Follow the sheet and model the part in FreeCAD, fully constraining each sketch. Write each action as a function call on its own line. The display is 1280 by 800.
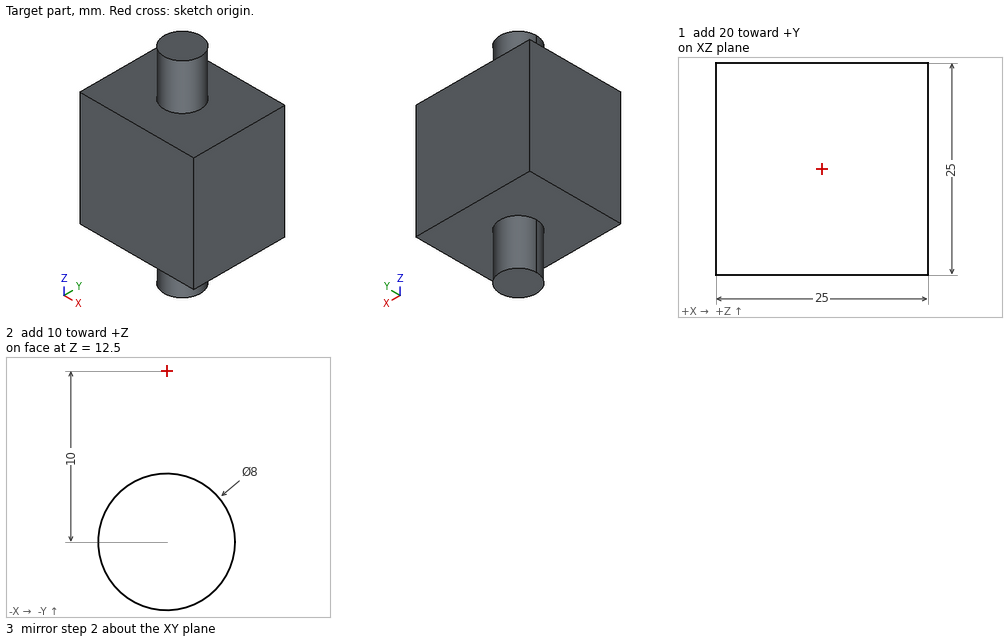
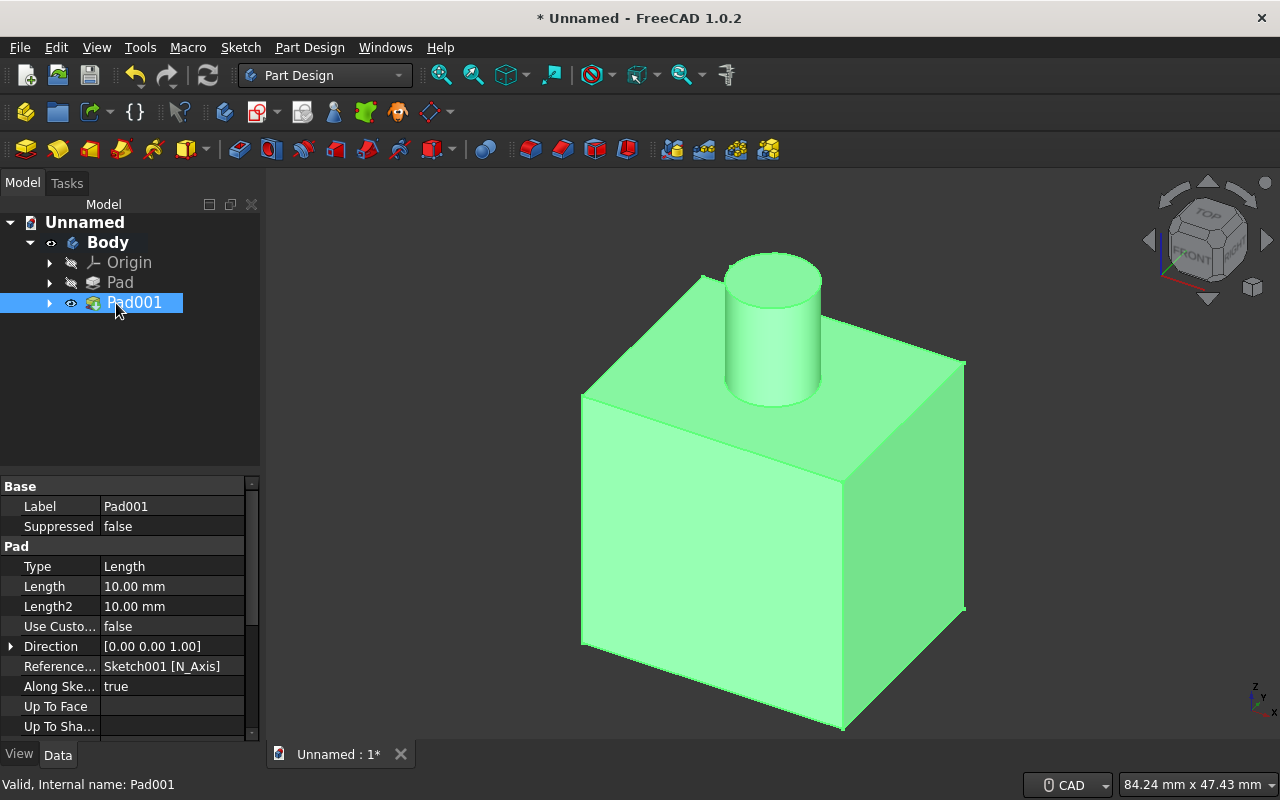
click(672, 150)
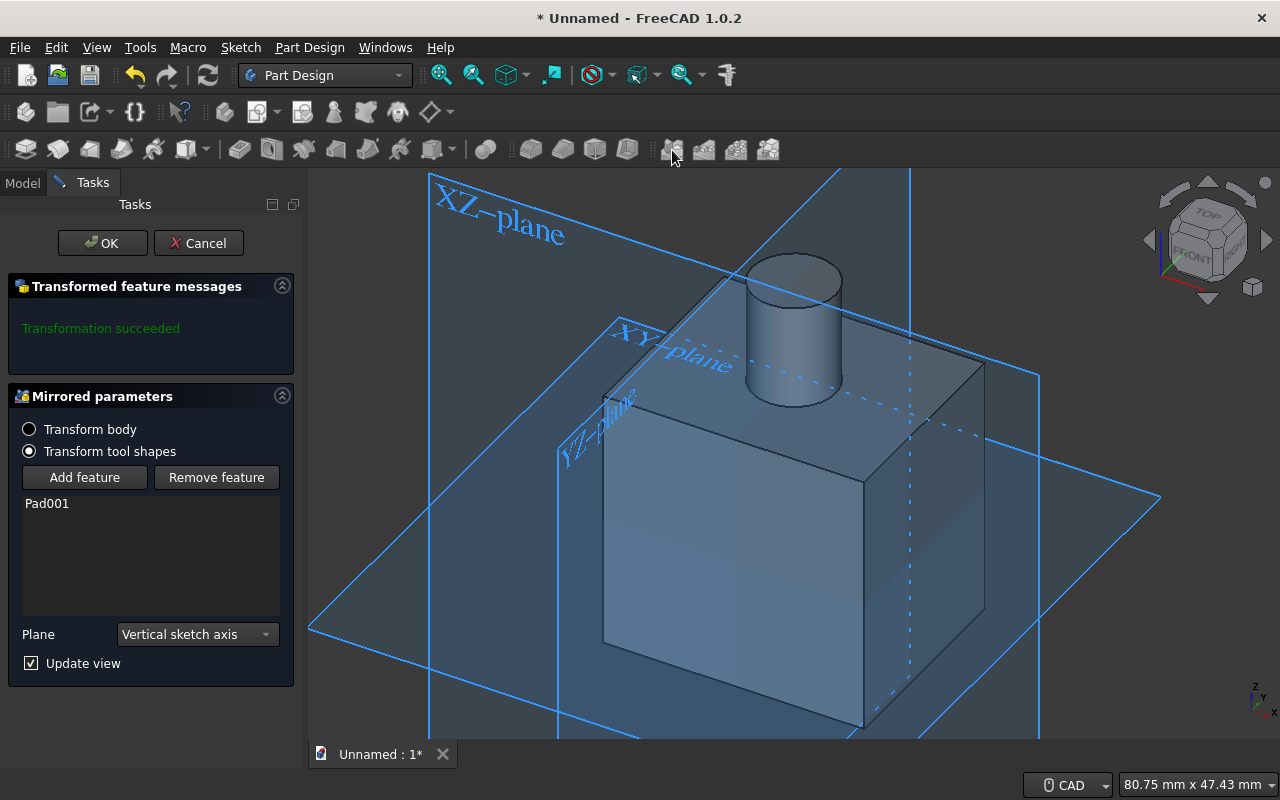
click(198, 634)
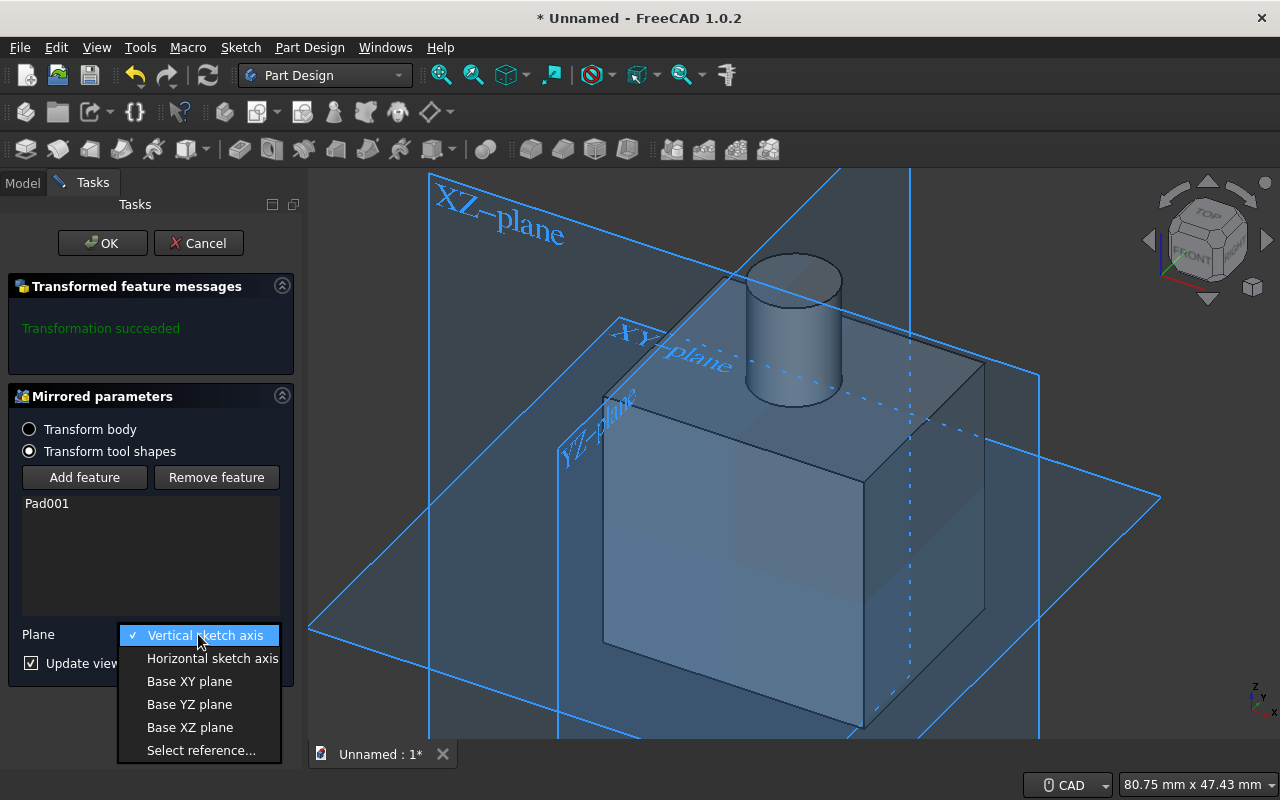
click(198, 682)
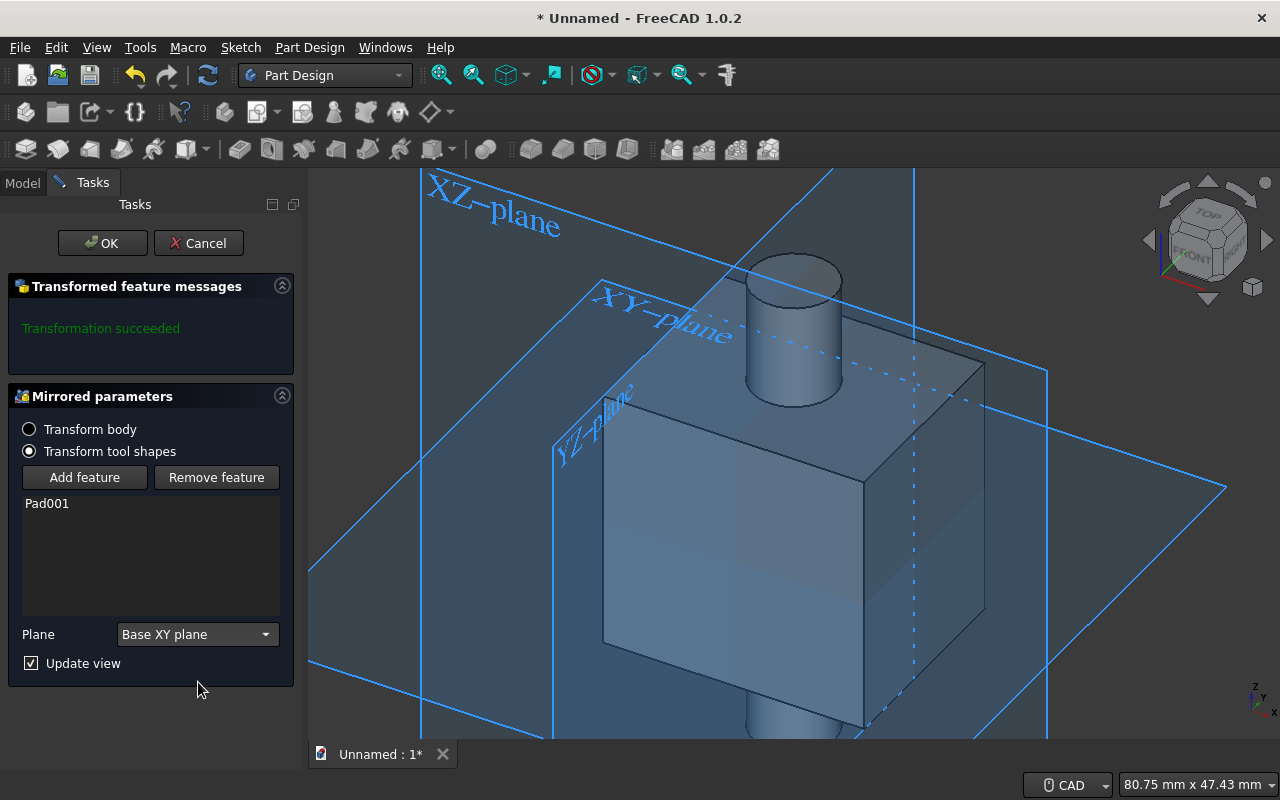
click(103, 243)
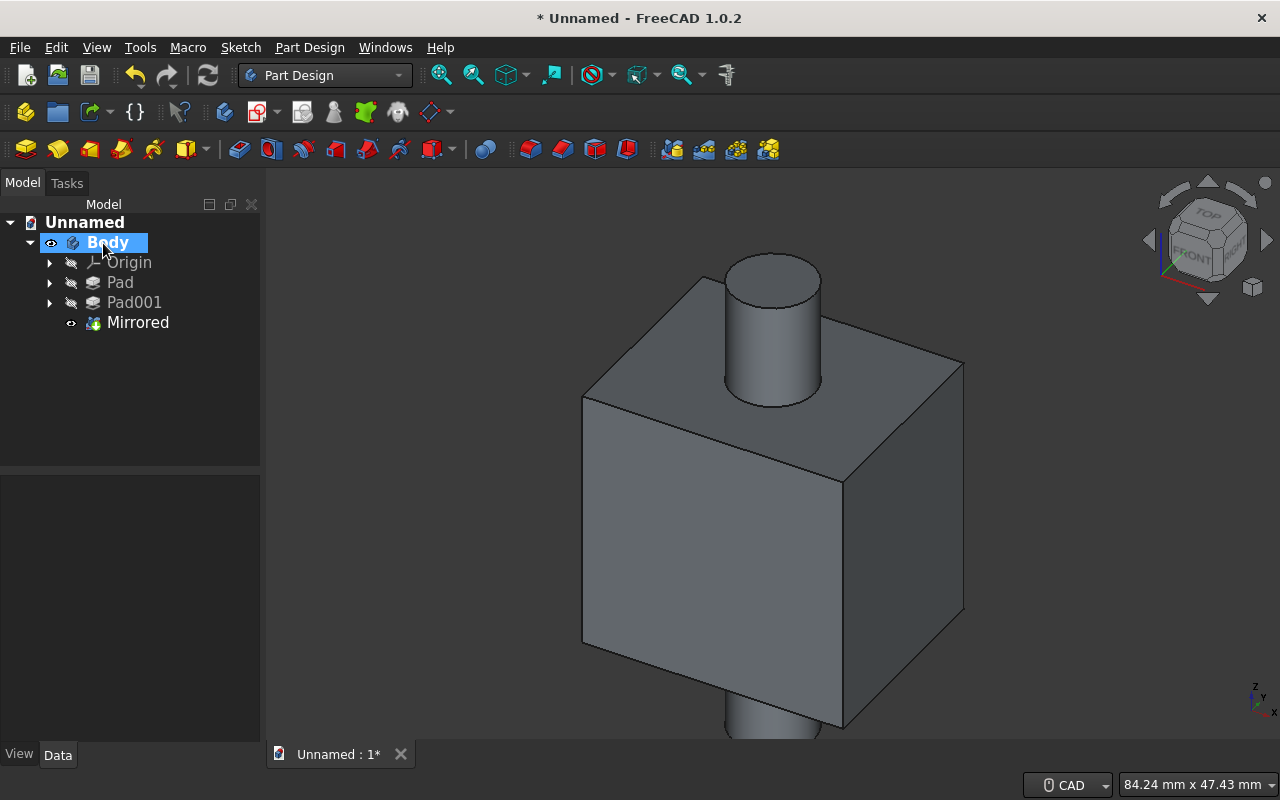
key(0)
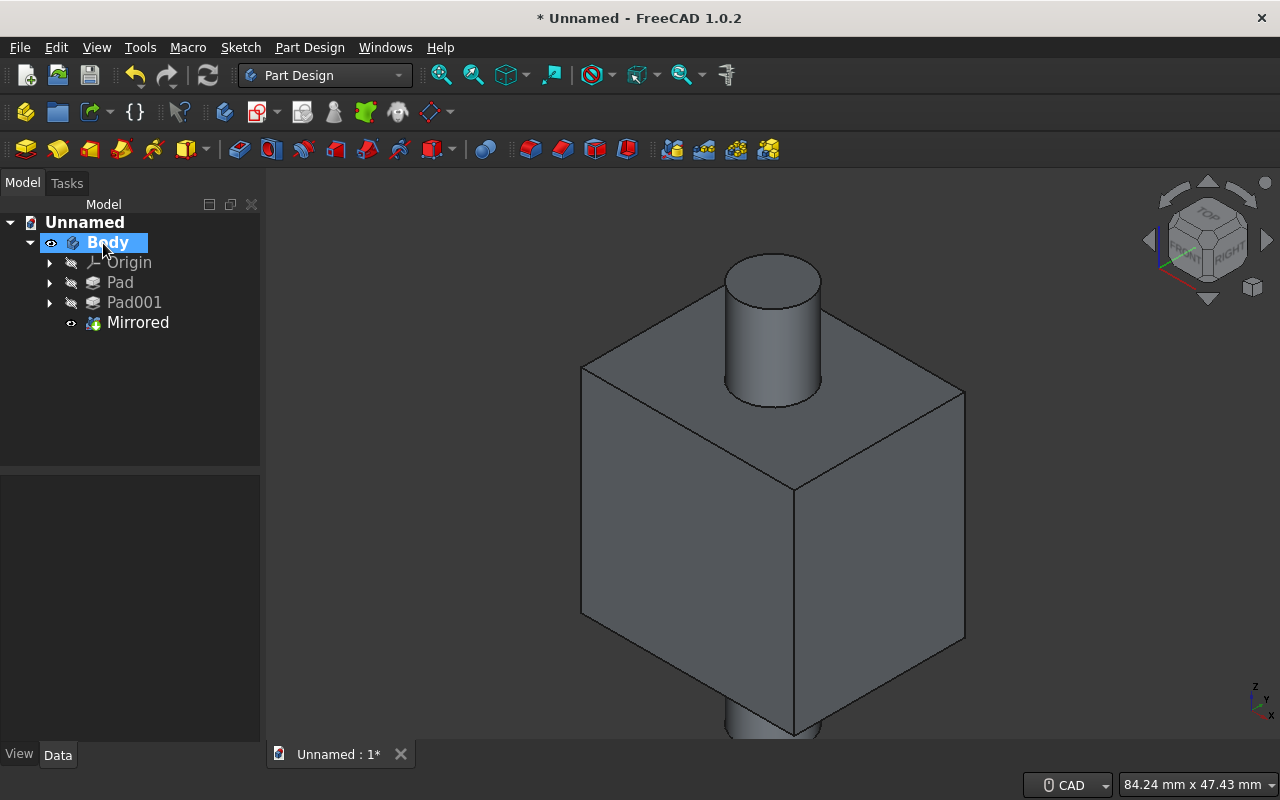
key(v)
key(f)